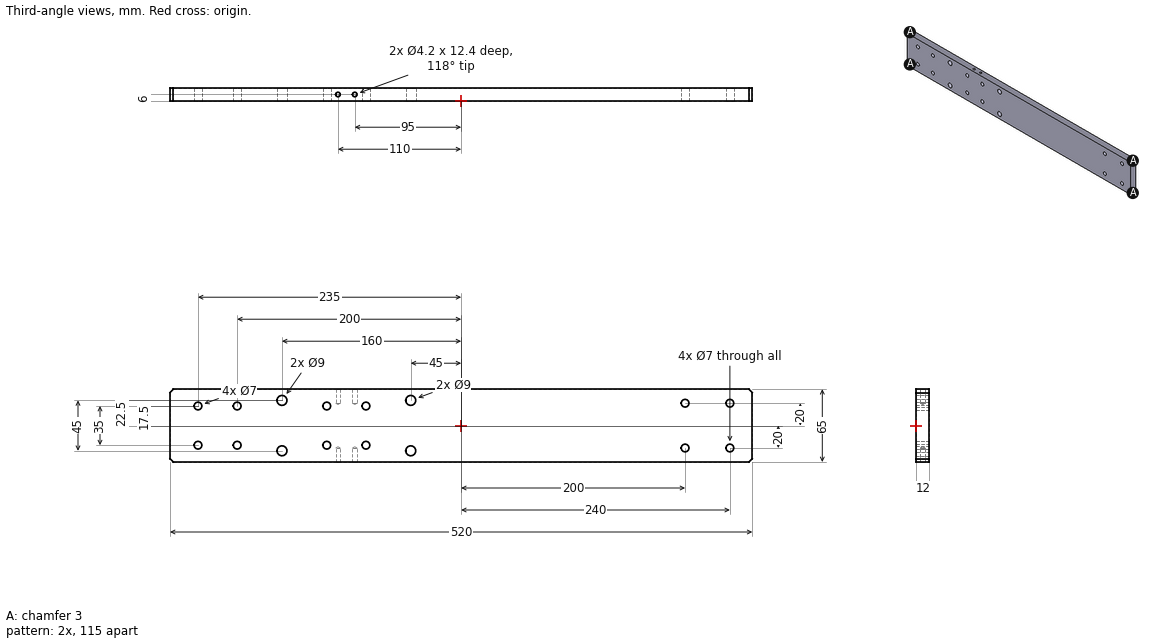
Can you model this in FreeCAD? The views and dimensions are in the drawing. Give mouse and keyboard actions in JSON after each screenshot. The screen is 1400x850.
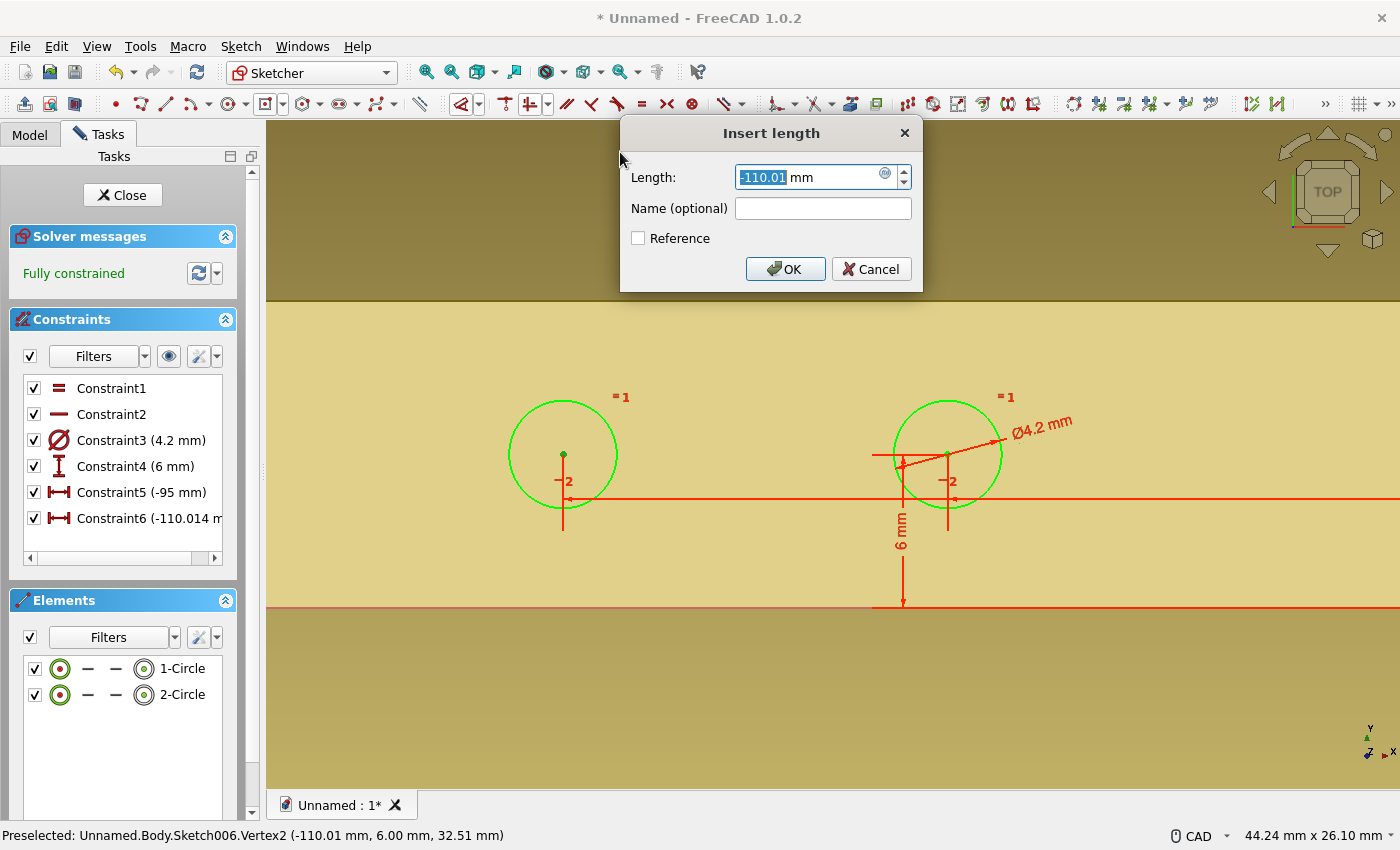
{"action": "type", "text": "-110"}
{"action": "key", "text": "Return"}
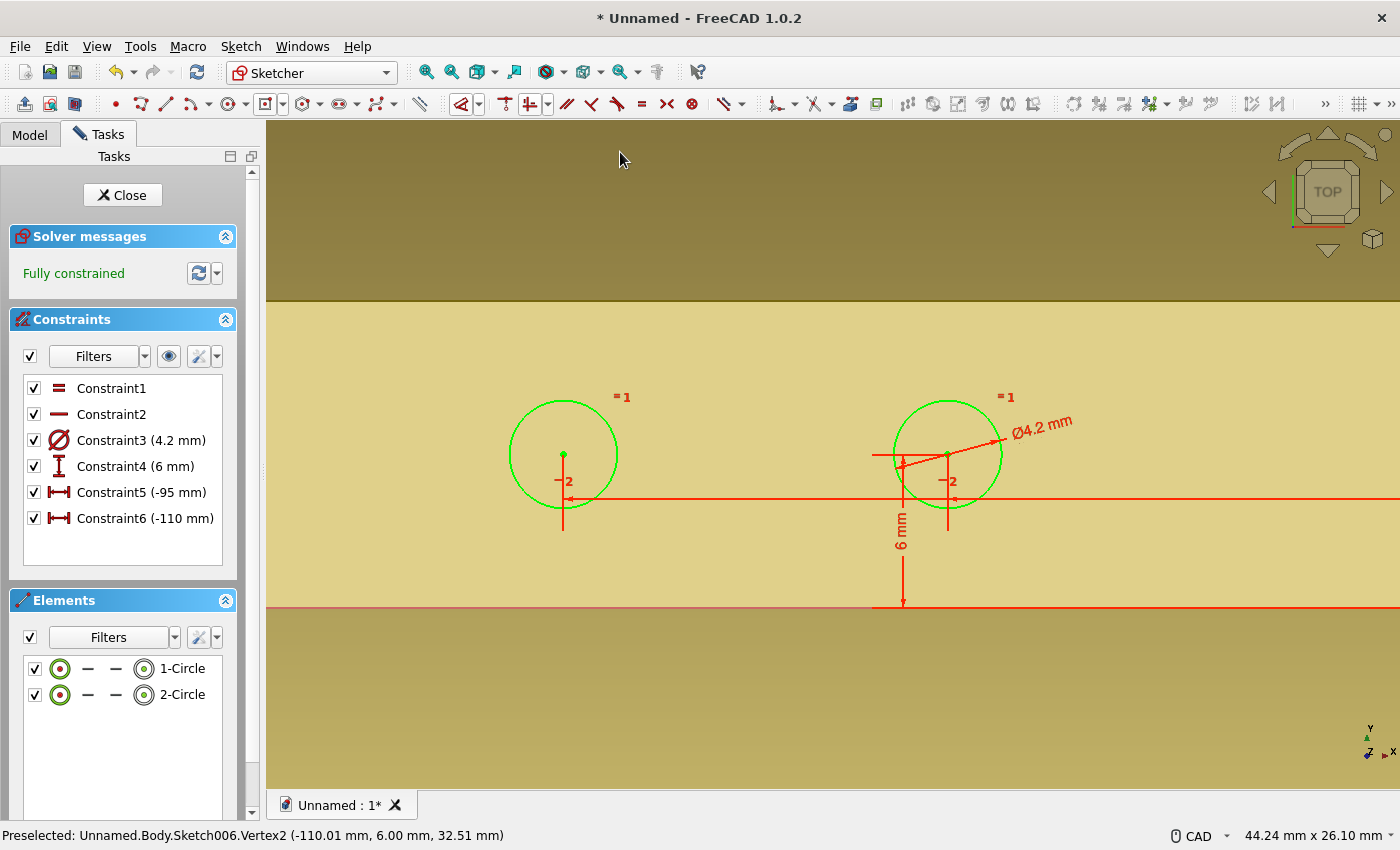
{"action": "left_click", "coordinate": [123, 195]}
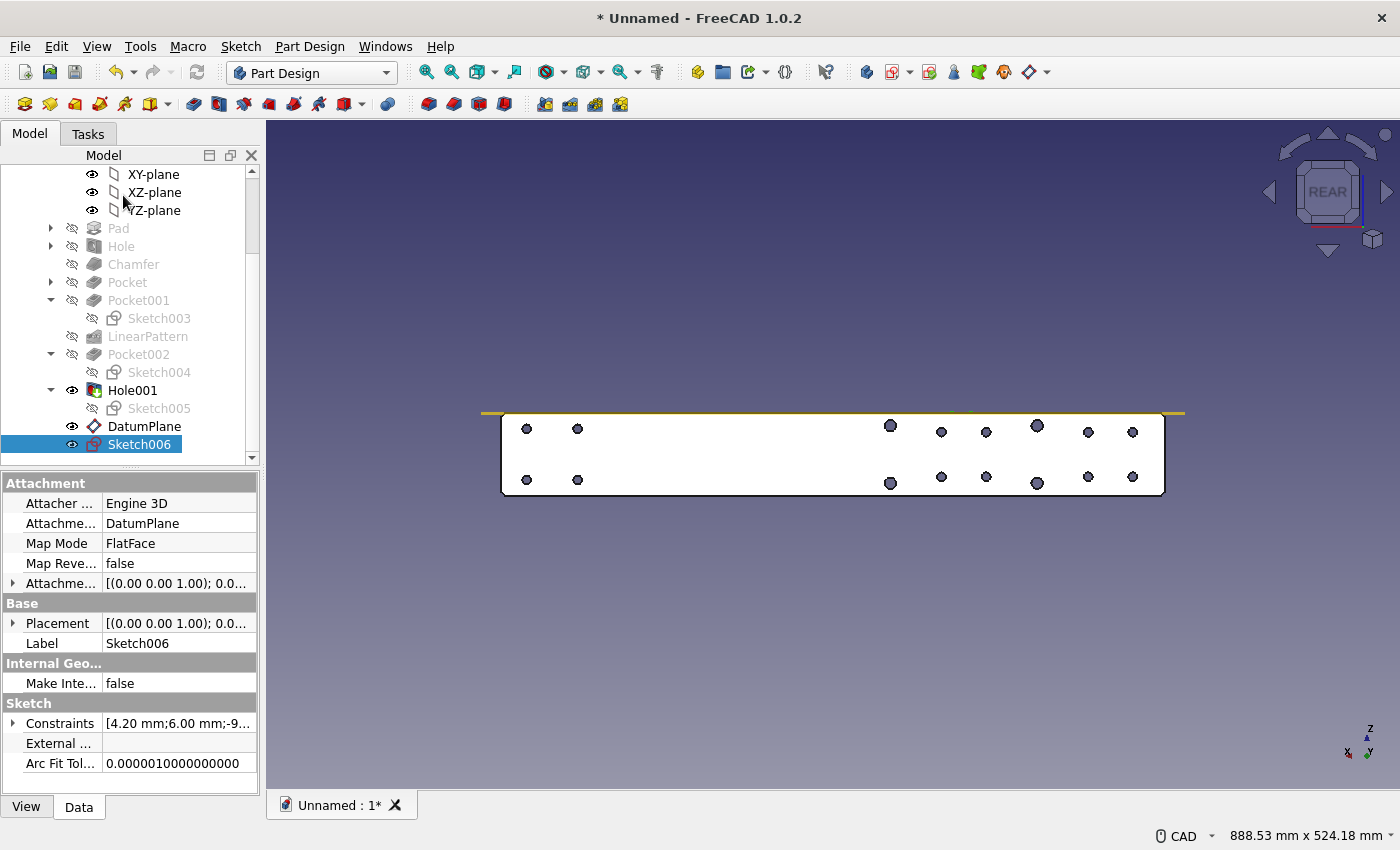
{"action": "left_click", "coordinate": [219, 104]}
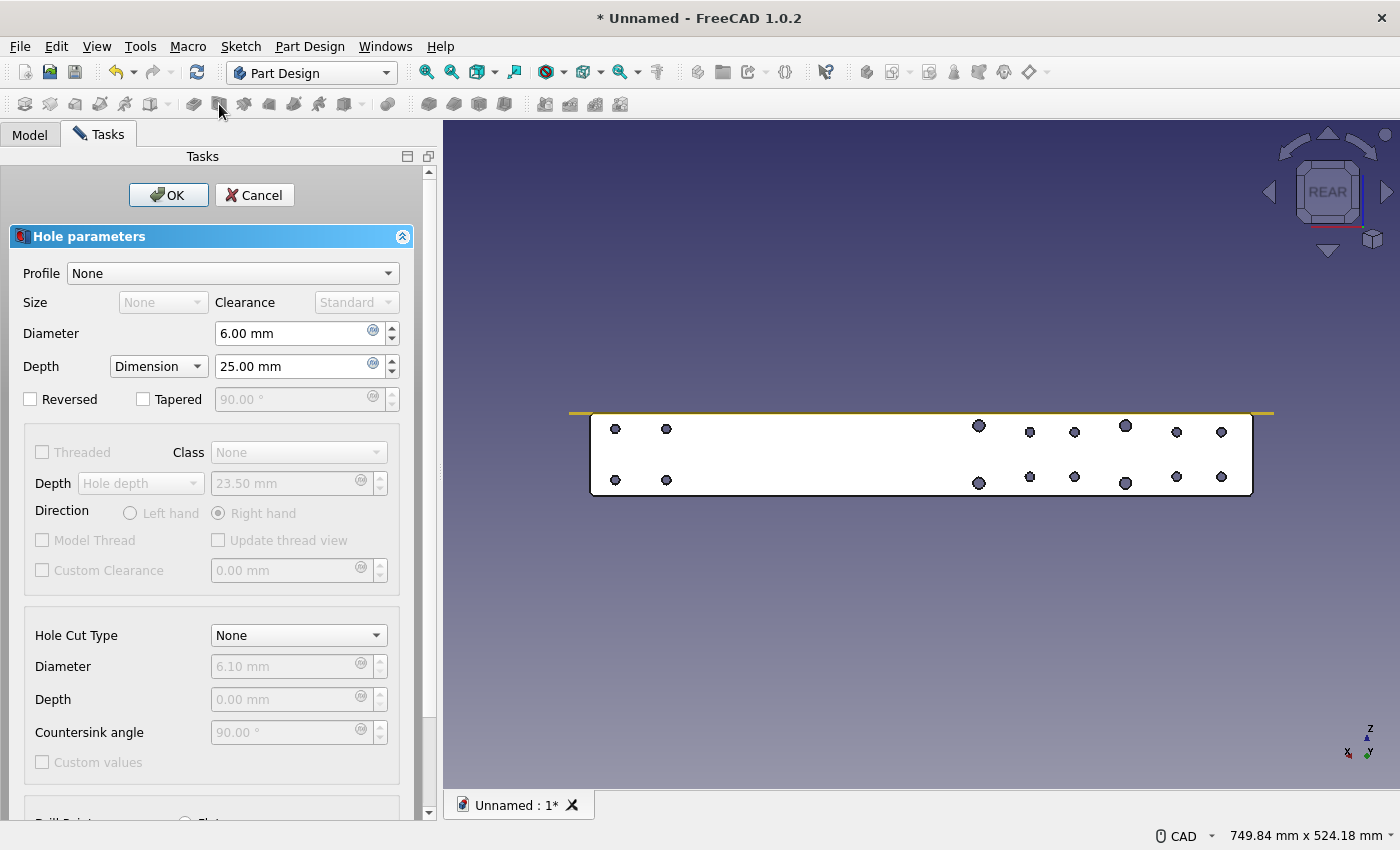
{"action": "triple_click", "coordinate": [300, 334]}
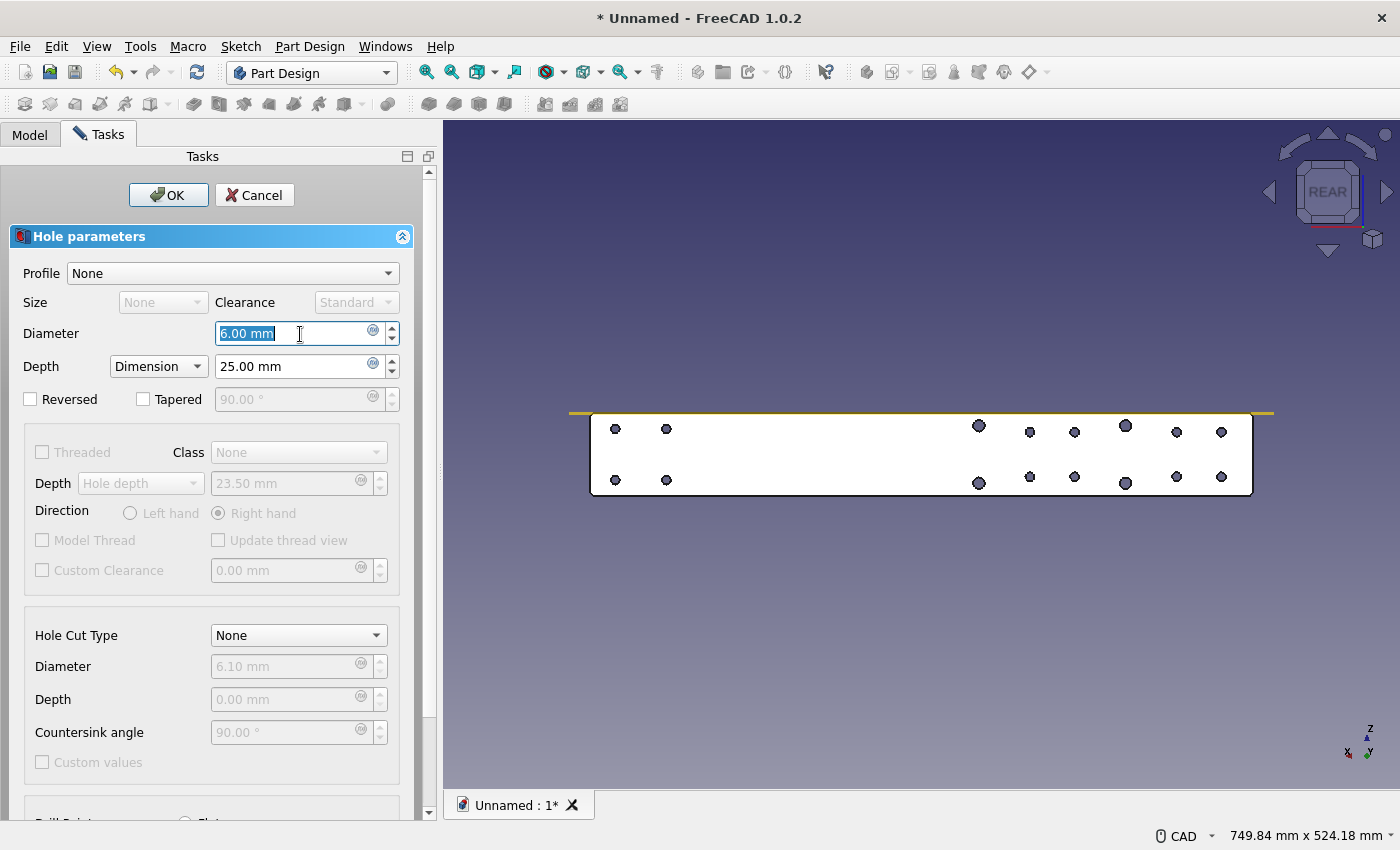
{"action": "type", "text": "4.2"}
{"action": "key", "text": "Tab"}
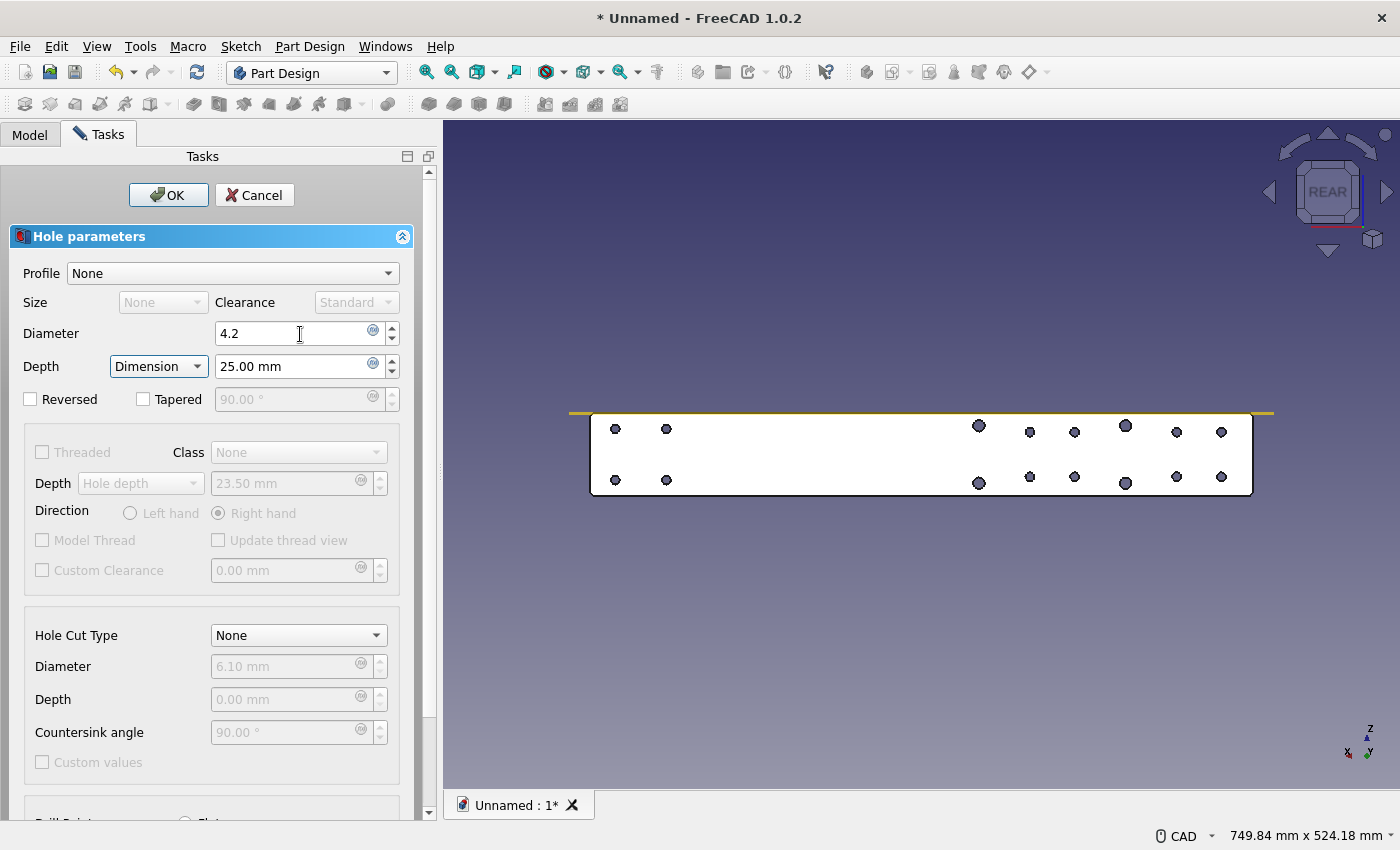
{"action": "triple_click", "coordinate": [300, 366]}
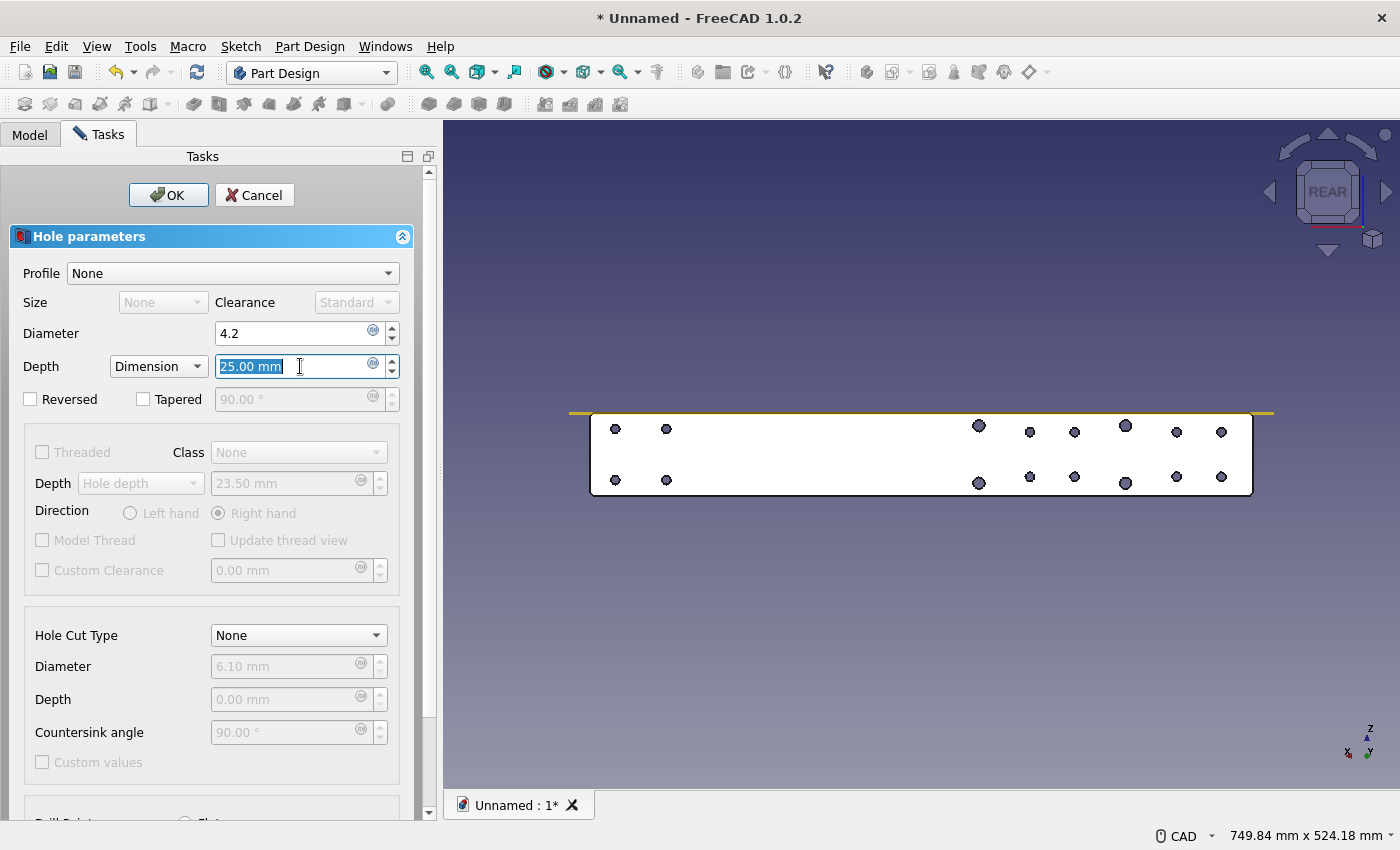
{"action": "type", "text": "12.4"}
{"action": "key", "text": "Tab"}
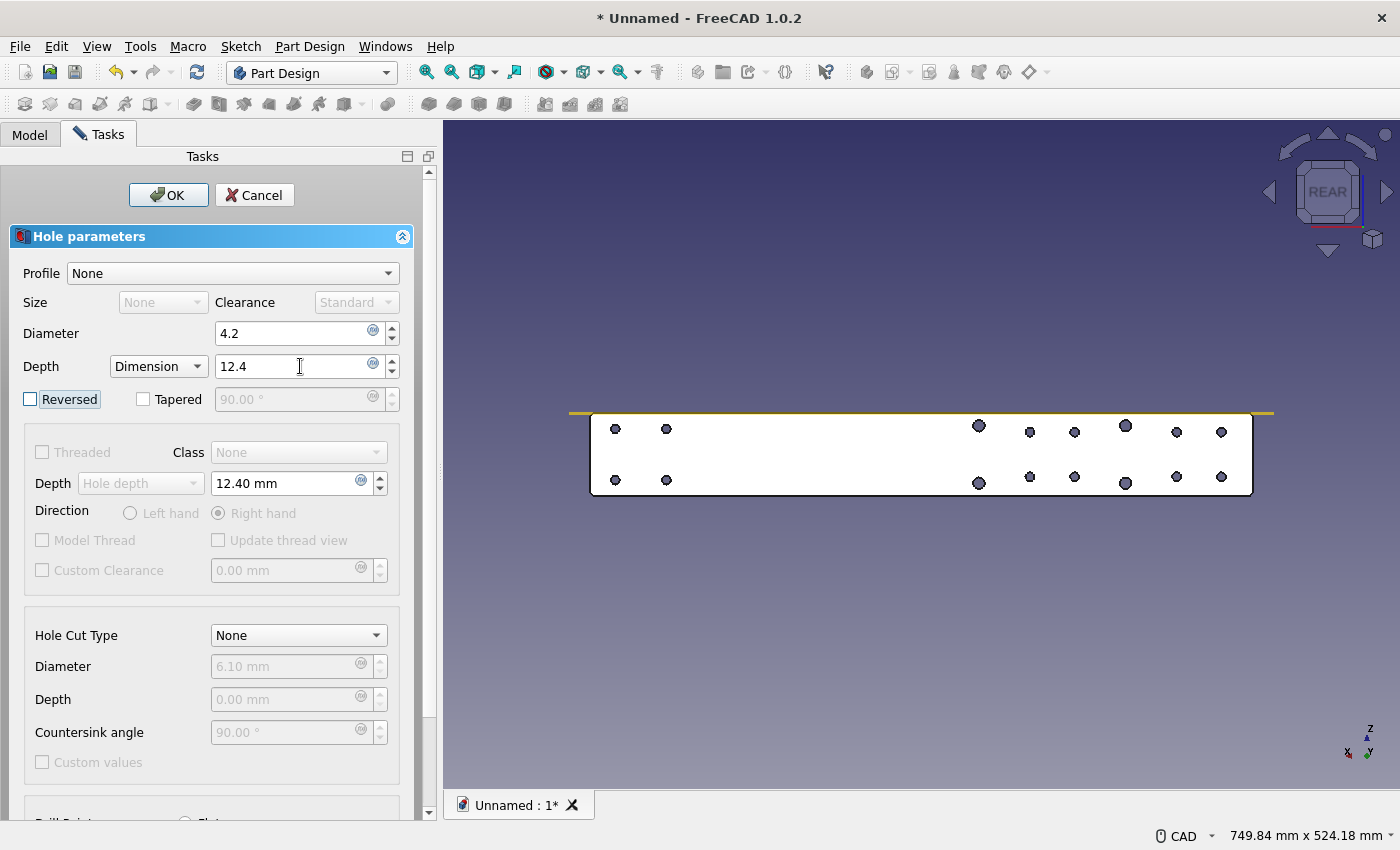
{"action": "left_click", "coordinate": [169, 195]}